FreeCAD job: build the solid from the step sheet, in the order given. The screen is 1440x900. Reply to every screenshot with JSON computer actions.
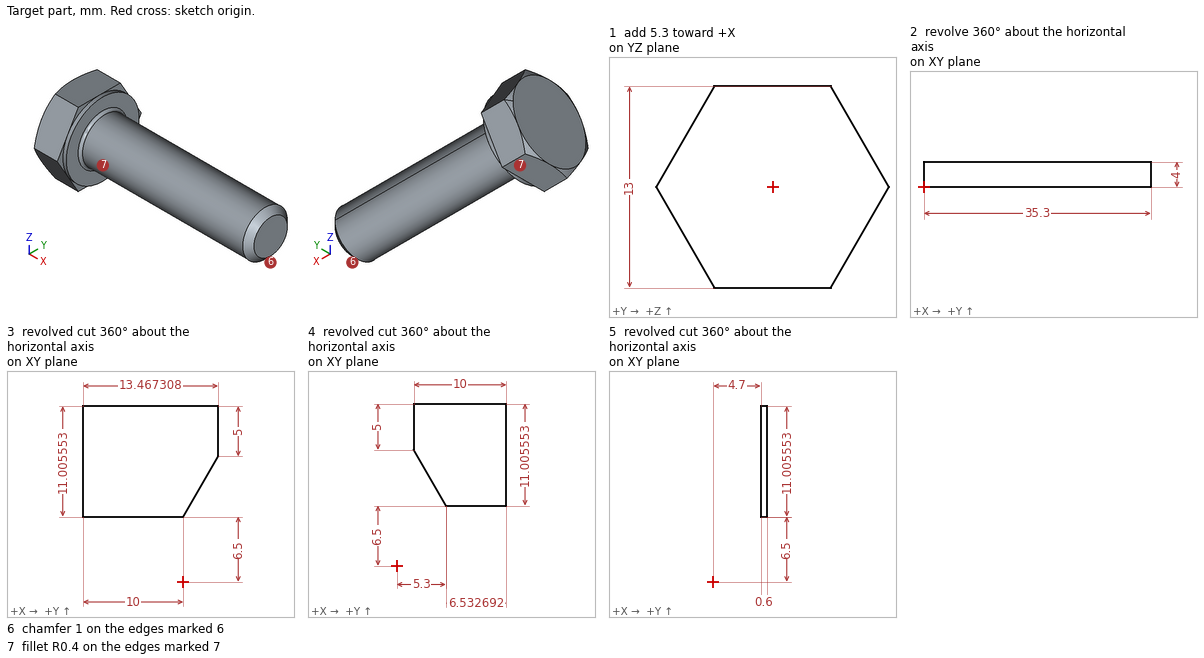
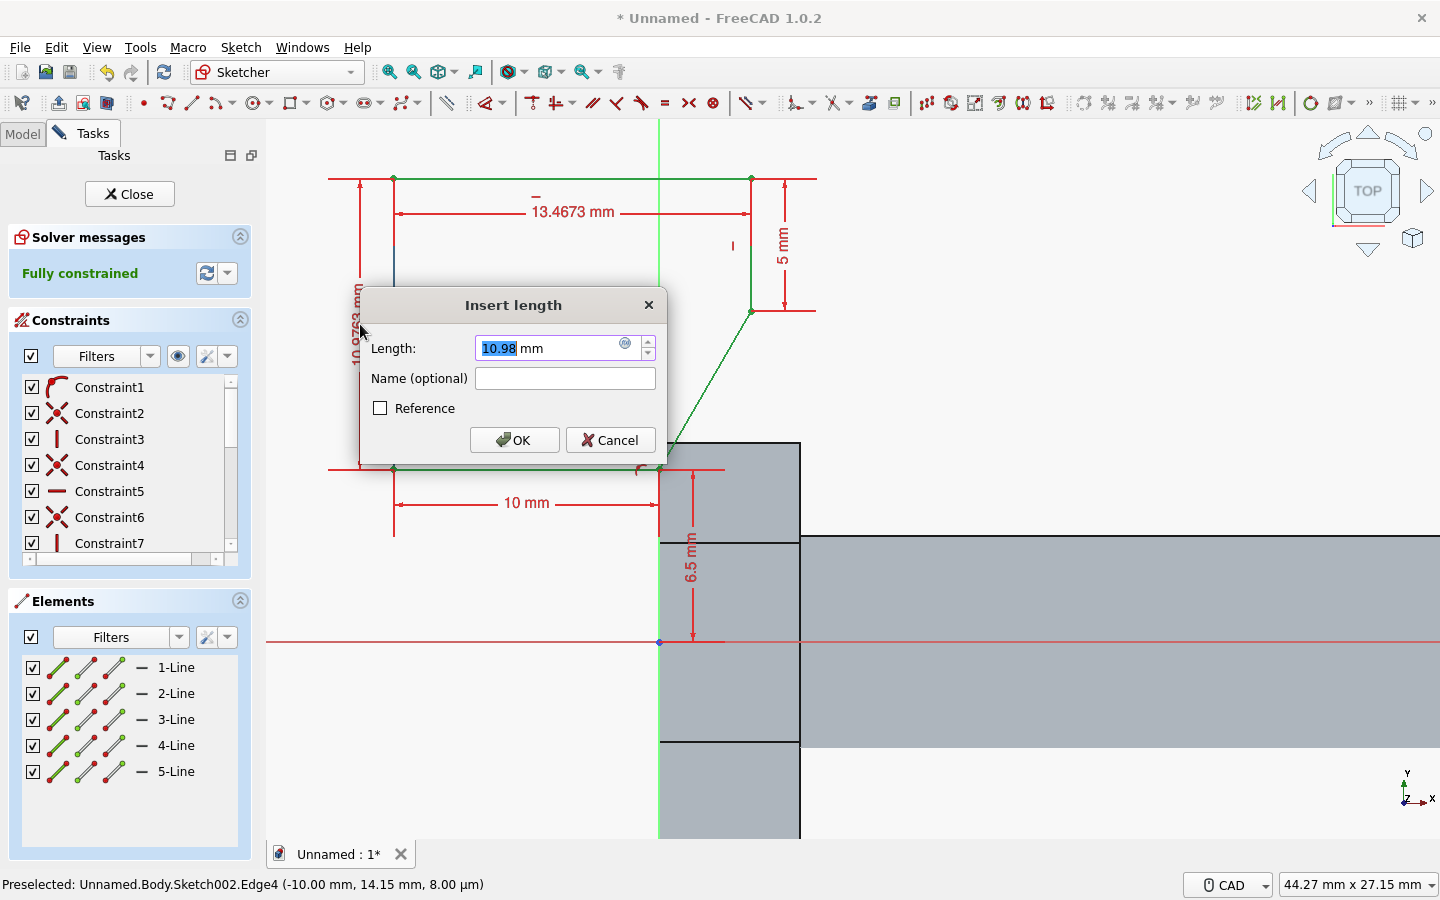
{"action": "type", "text": "11.005553"}
{"action": "key", "text": "Return"}
{"action": "key", "text": "Escape"}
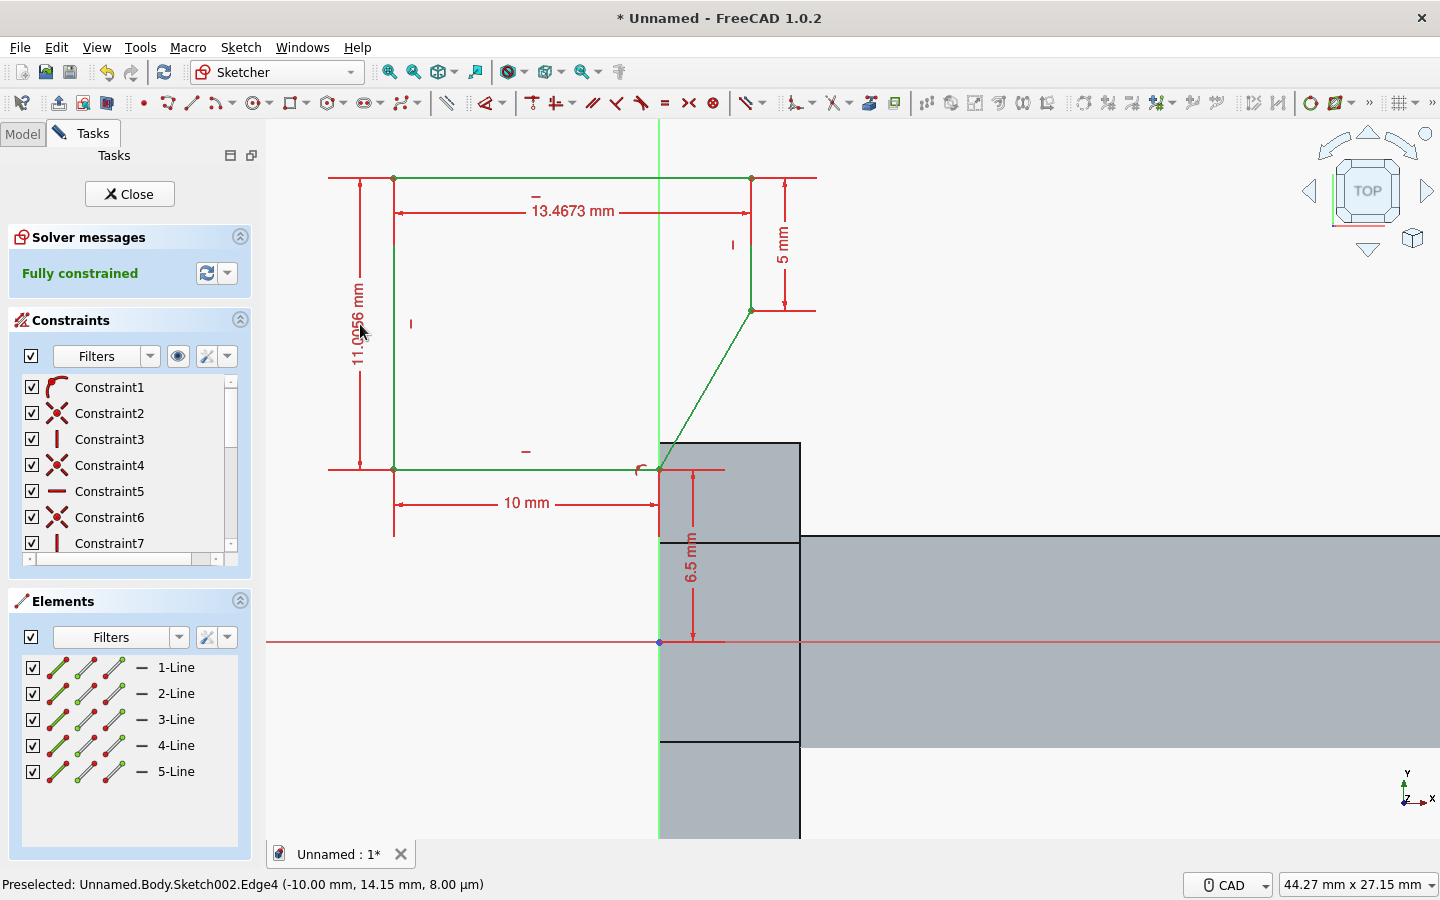
{"action": "left_click", "coordinate": [130, 194]}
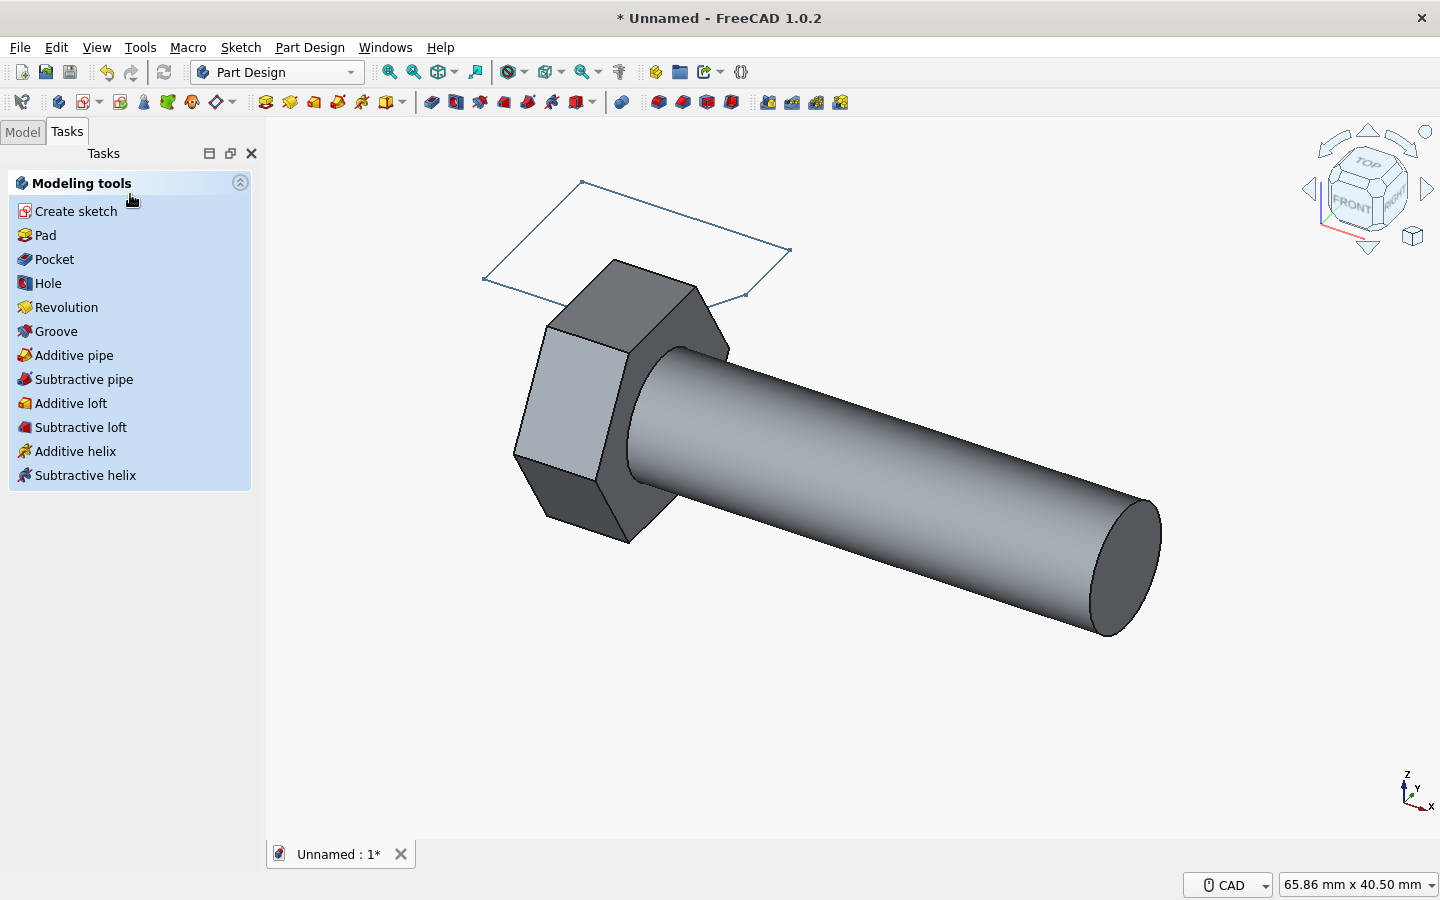
{"action": "left_click", "coordinate": [480, 102]}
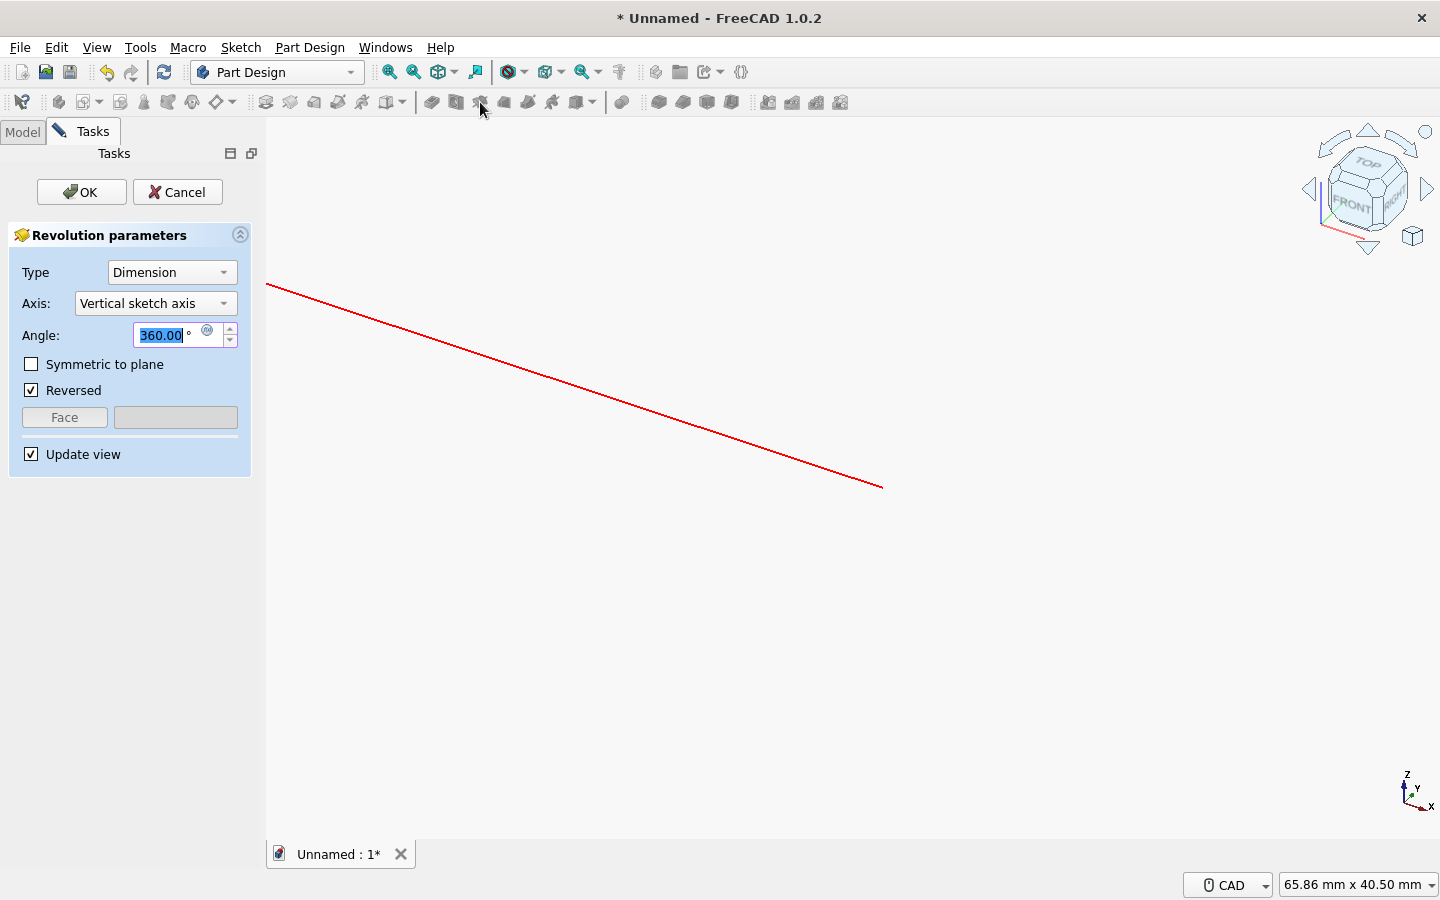
{"action": "left_click", "coordinate": [156, 304]}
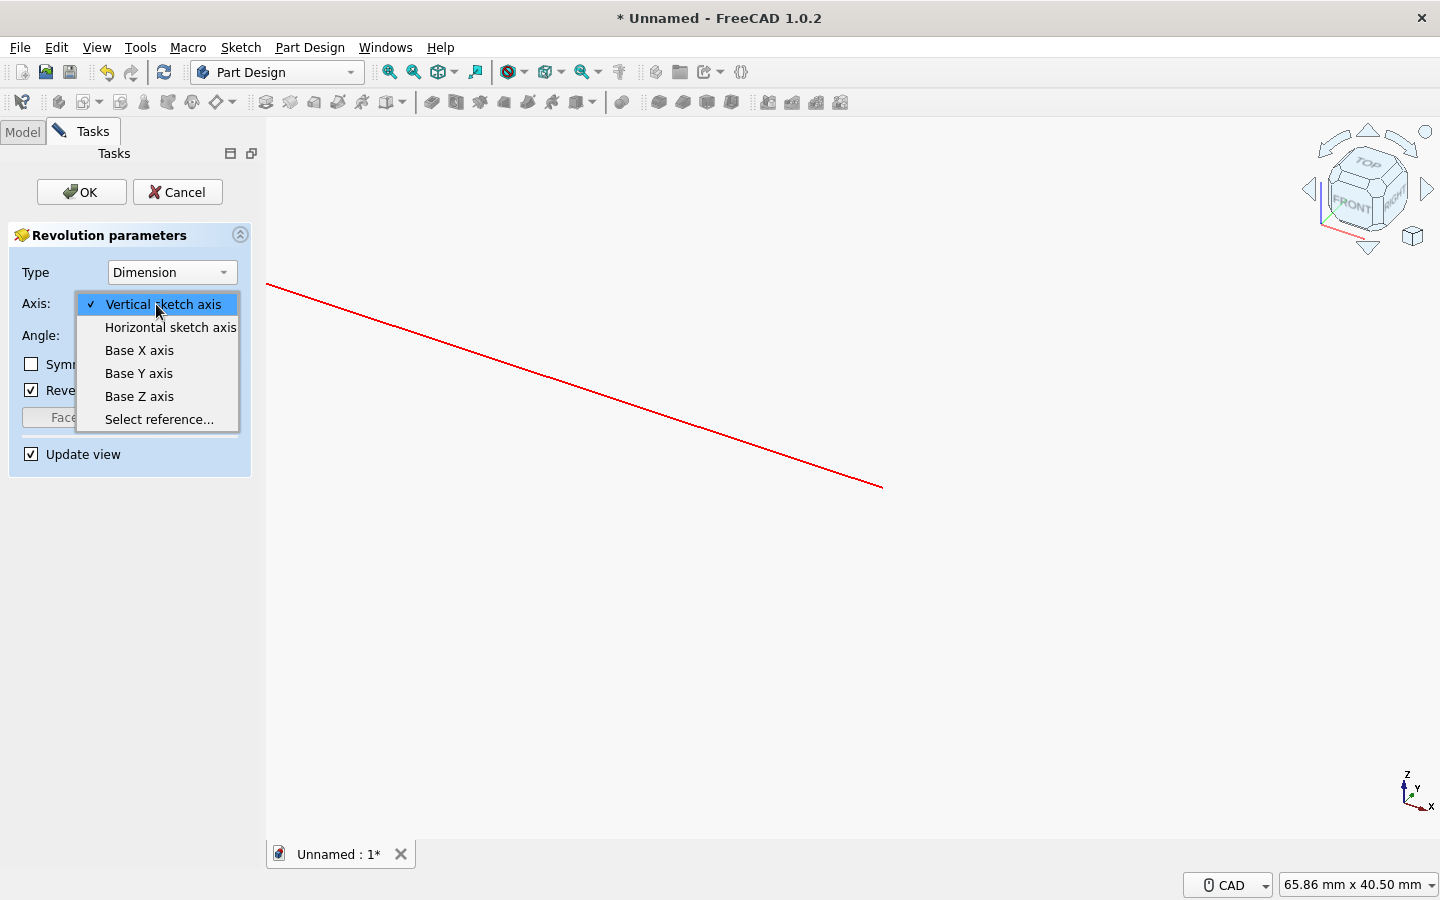
{"action": "left_click", "coordinate": [156, 328]}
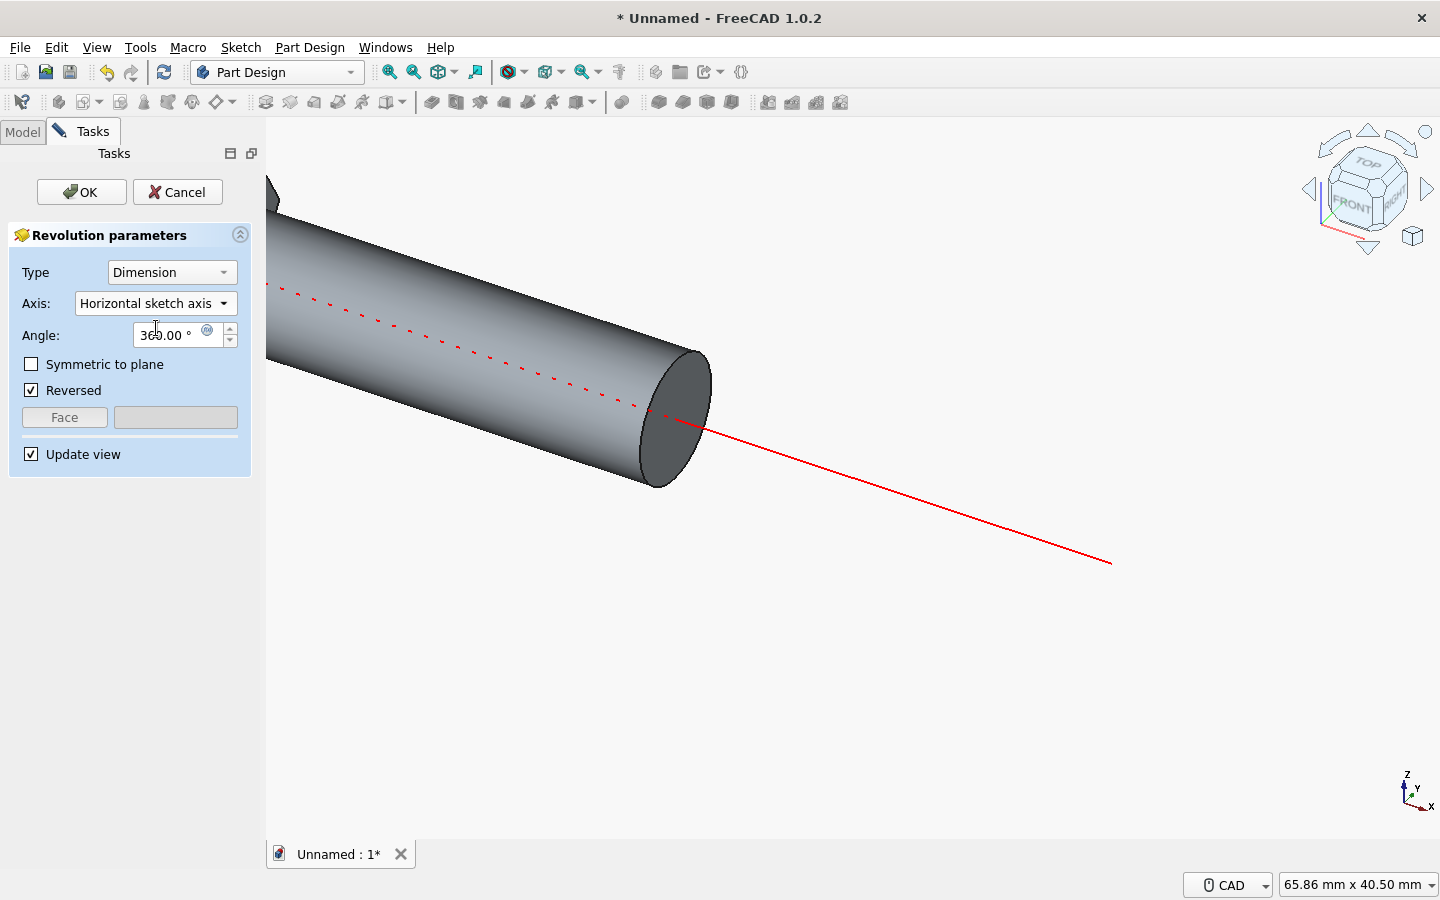
{"action": "left_click", "coordinate": [82, 192]}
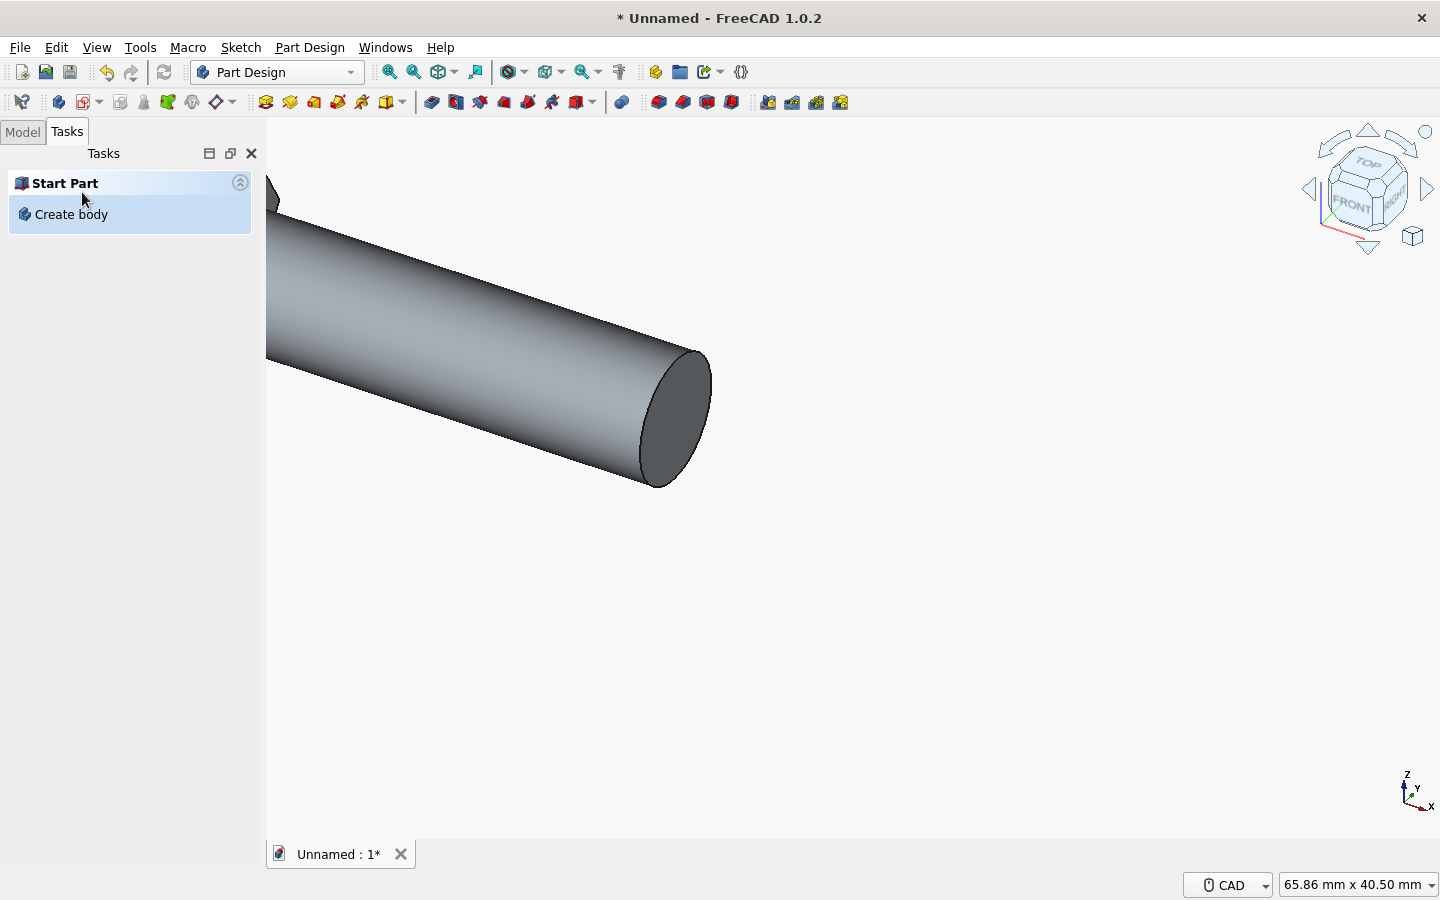
{"action": "key", "text": "v f"}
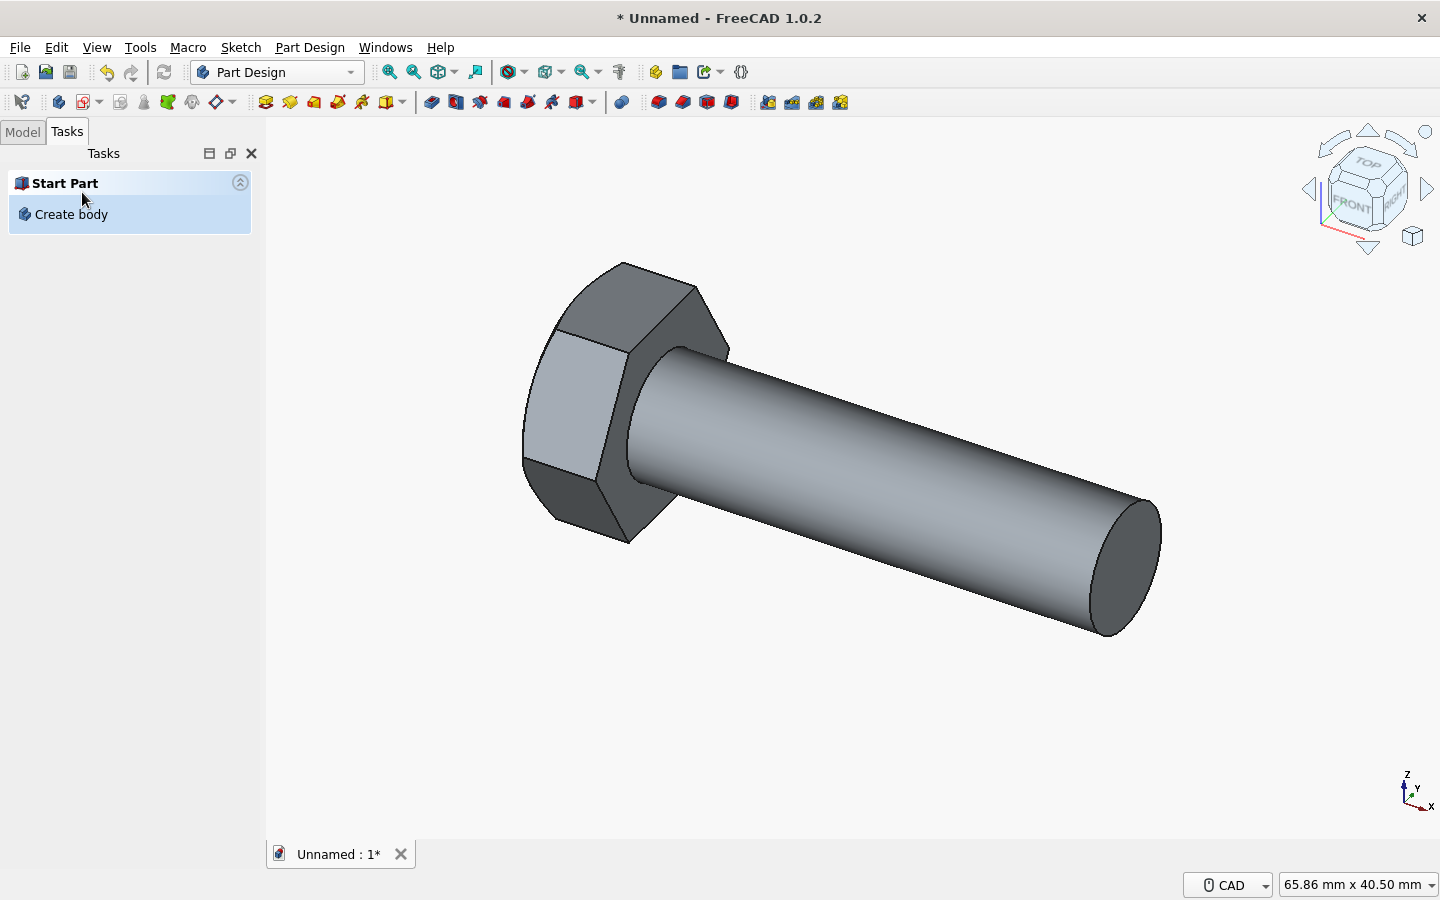
{"action": "left_click", "coordinate": [84, 102]}